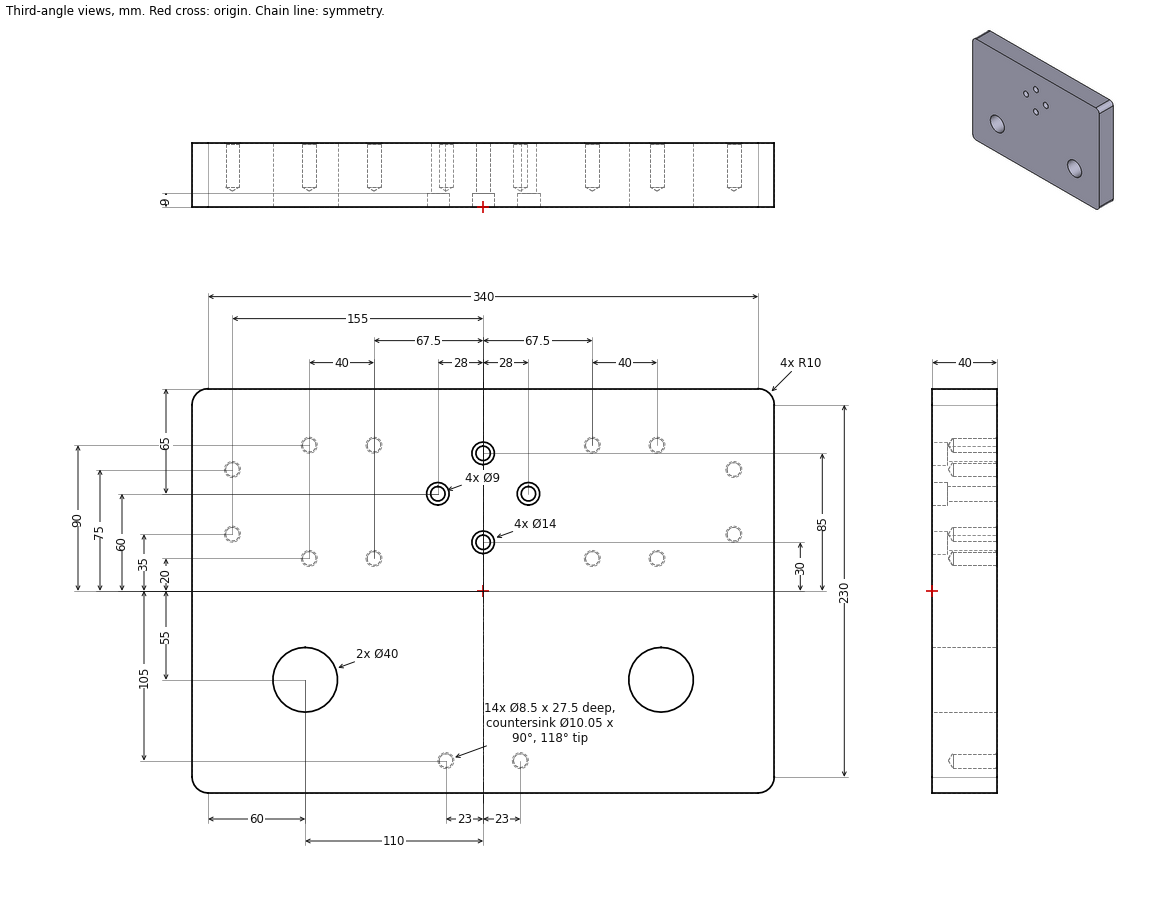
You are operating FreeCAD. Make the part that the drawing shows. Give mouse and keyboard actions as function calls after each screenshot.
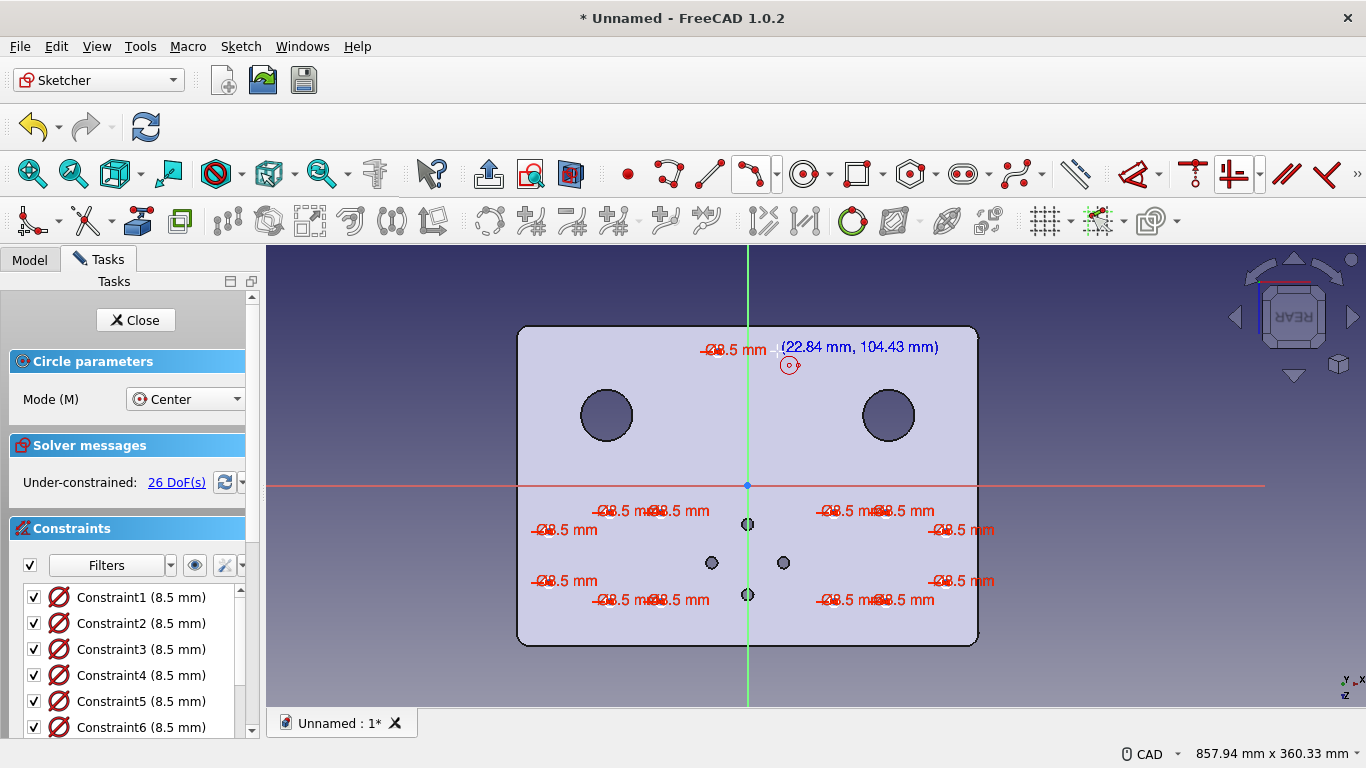
click(777, 351)
move(781, 347)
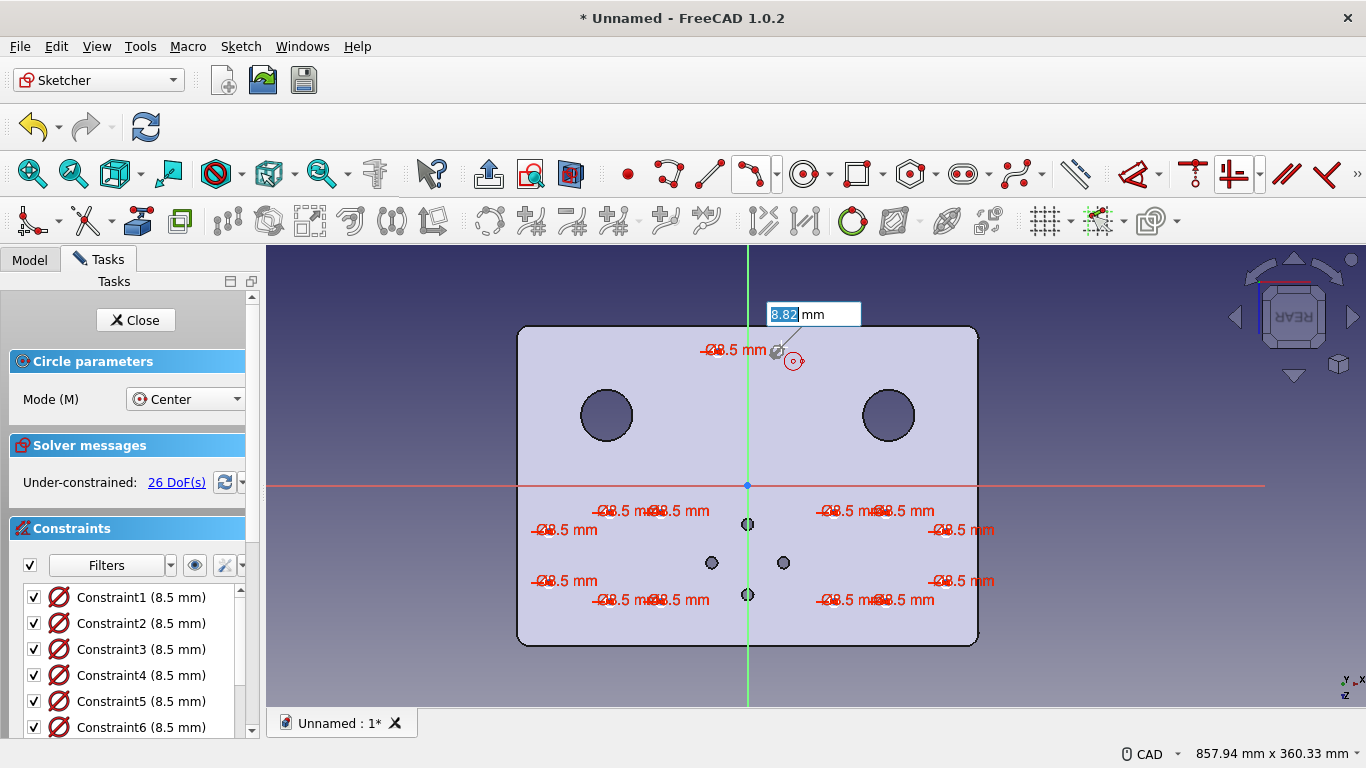
text(8.5)
key(Return)
key(Escape)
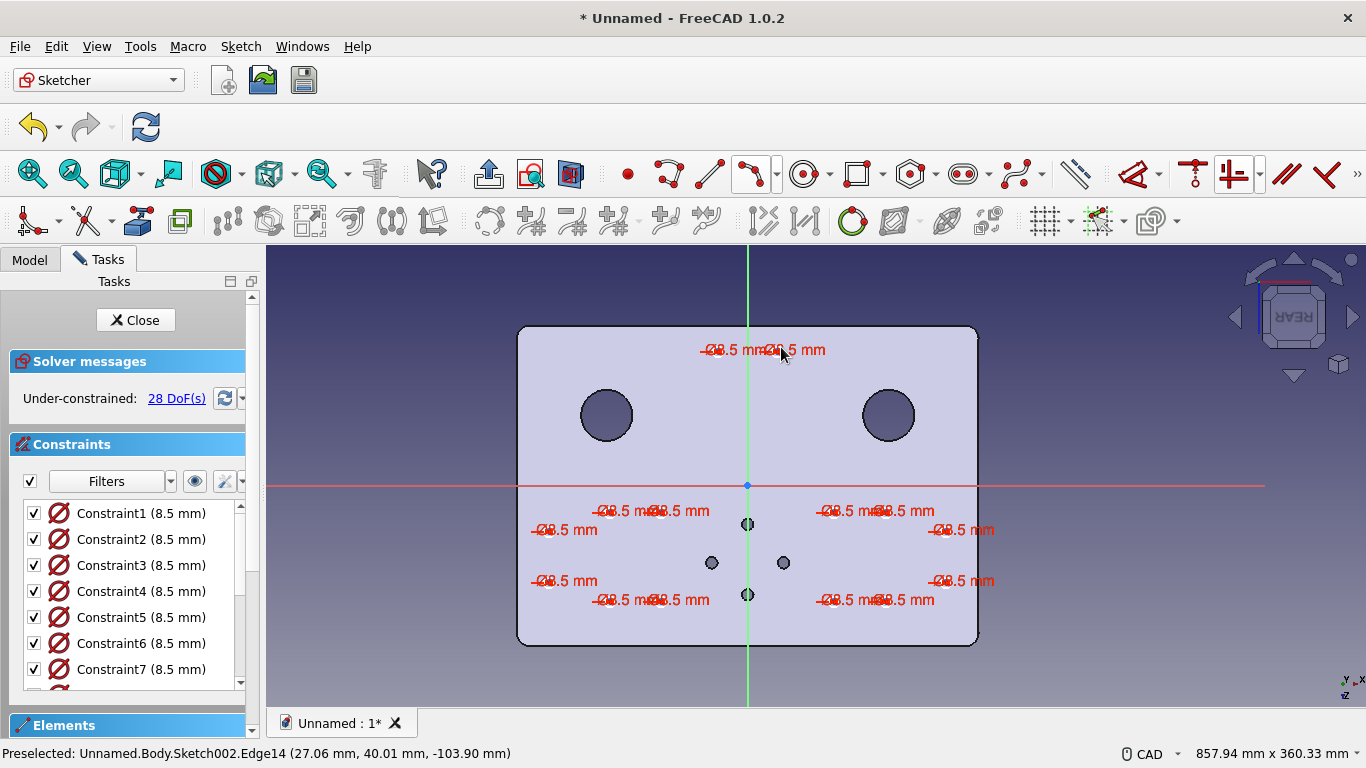
click(549, 532)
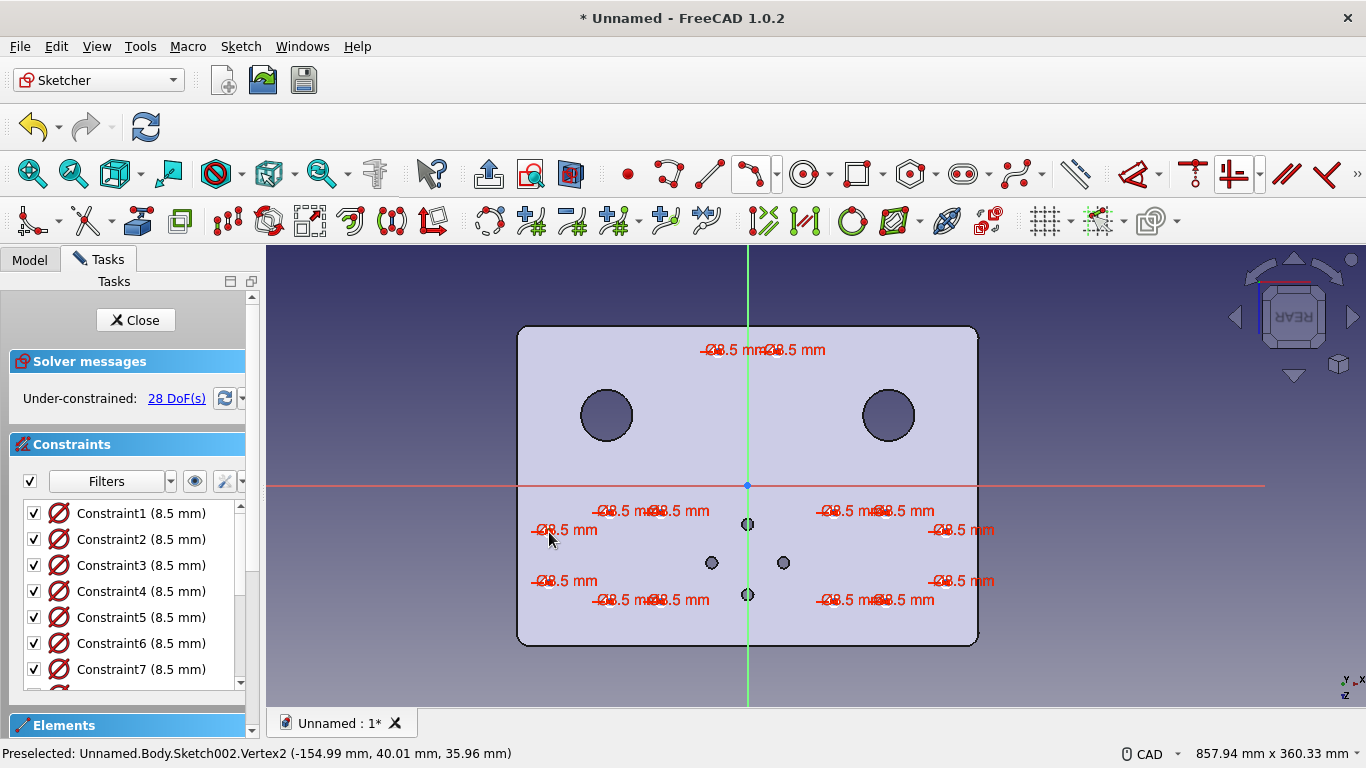
click(549, 583)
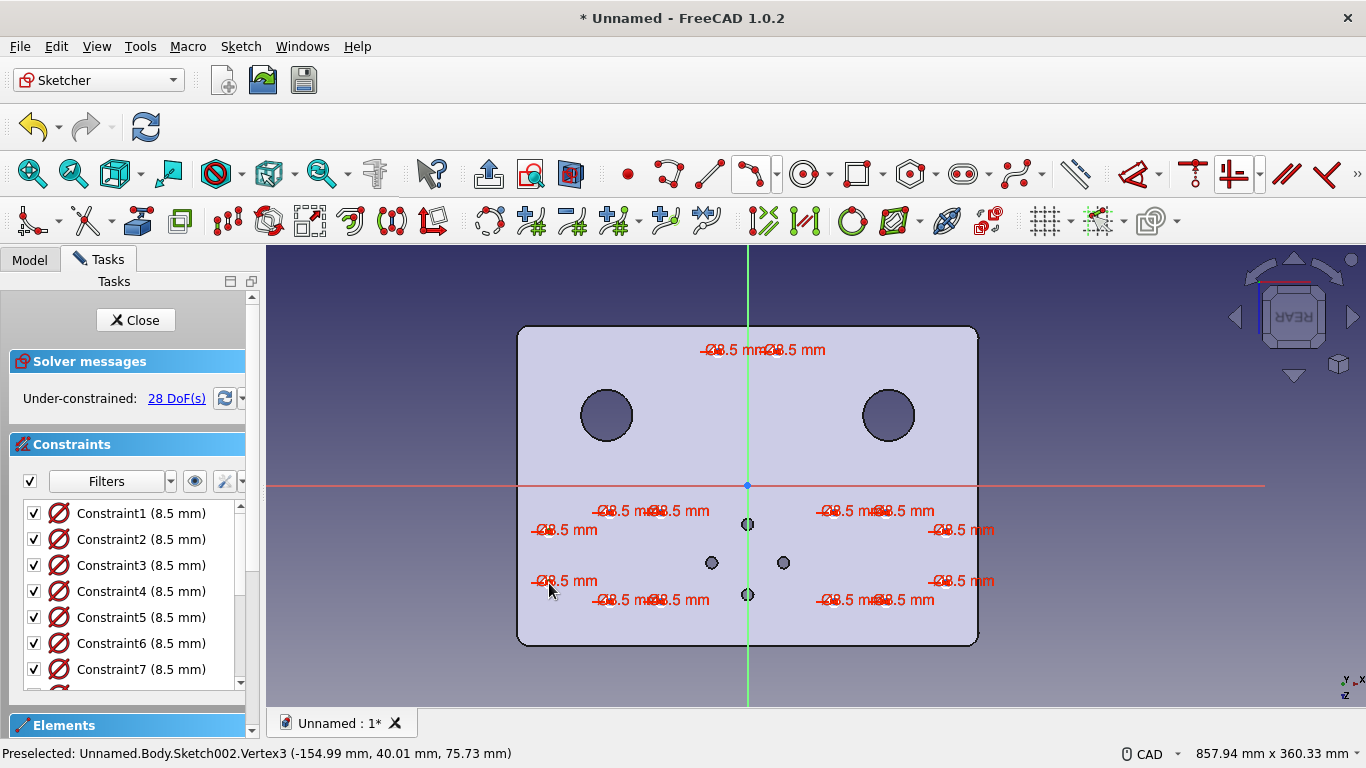
click(1260, 174)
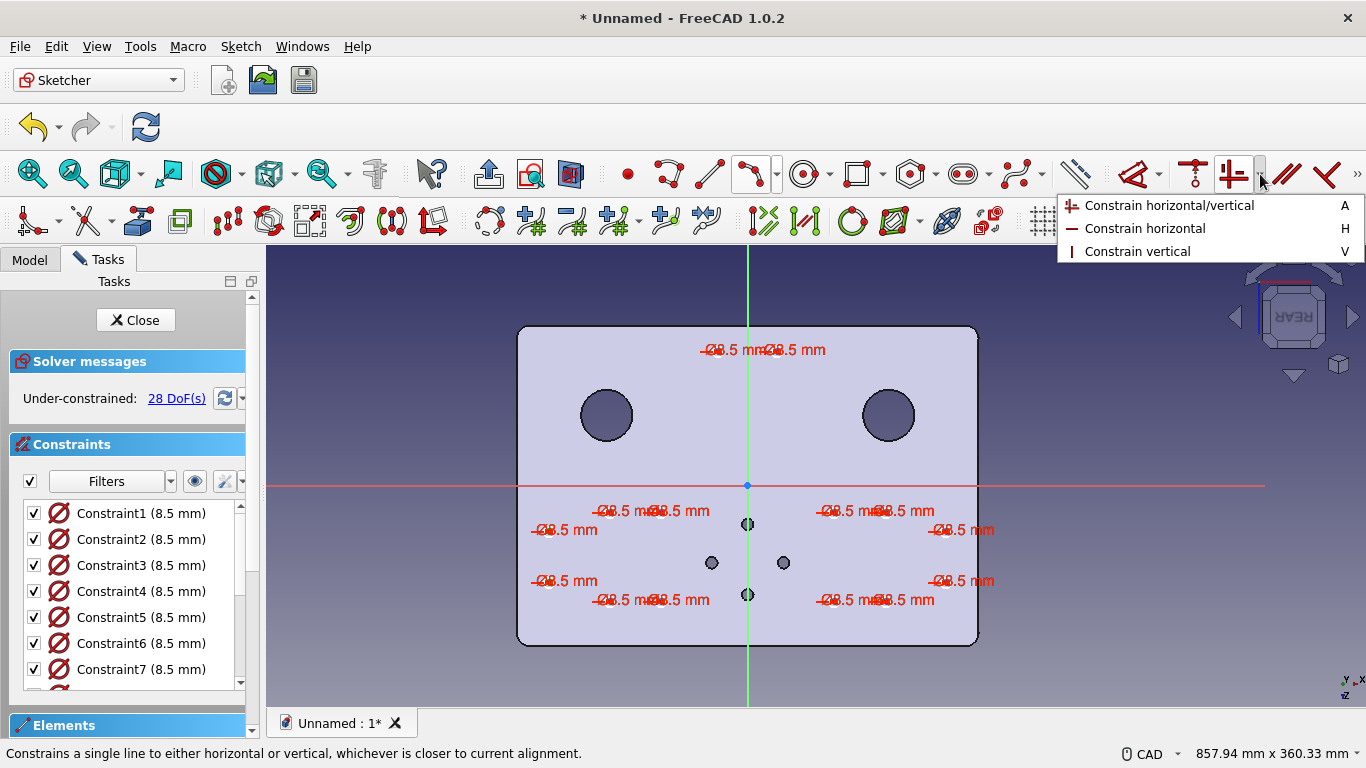
click(1211, 252)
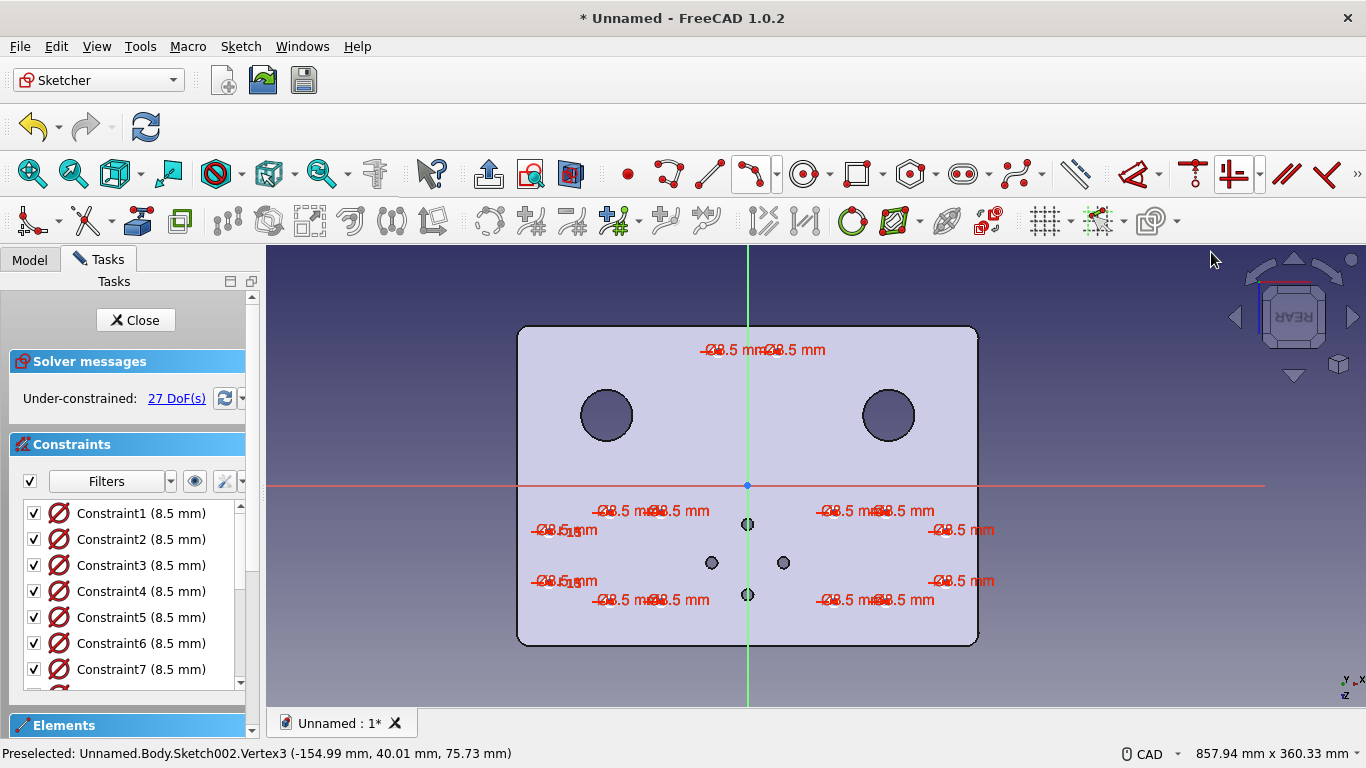
click(610, 513)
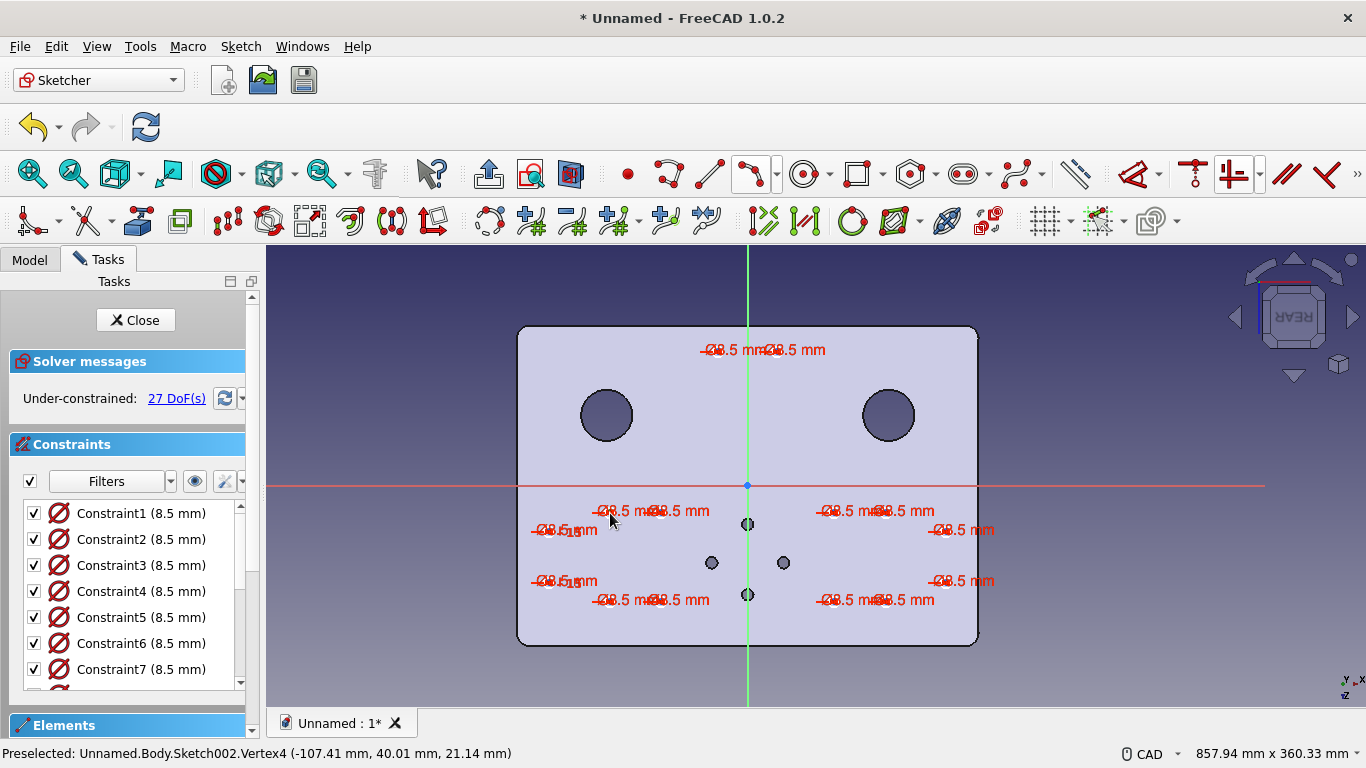
click(661, 513)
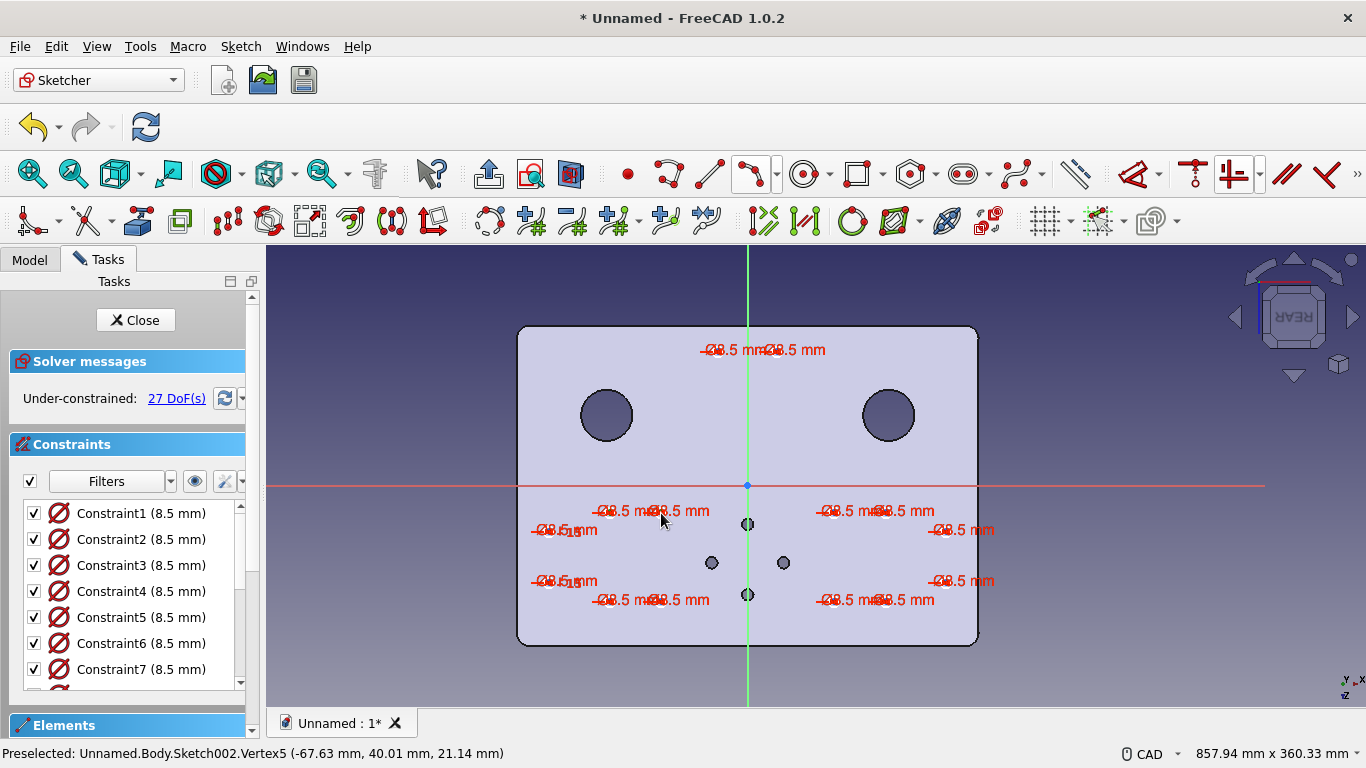
key(h)